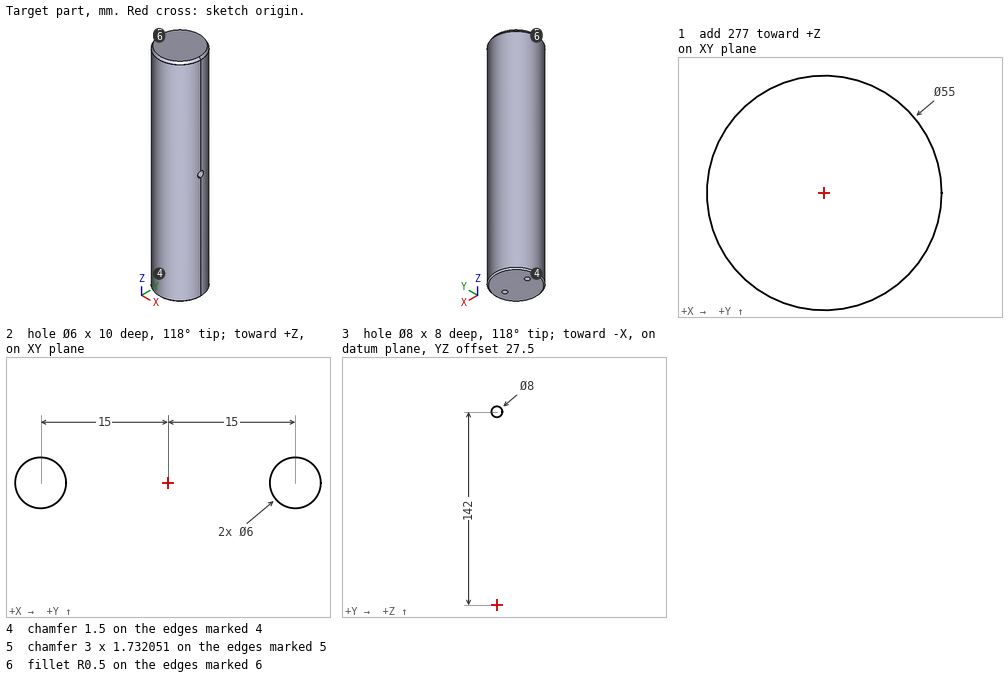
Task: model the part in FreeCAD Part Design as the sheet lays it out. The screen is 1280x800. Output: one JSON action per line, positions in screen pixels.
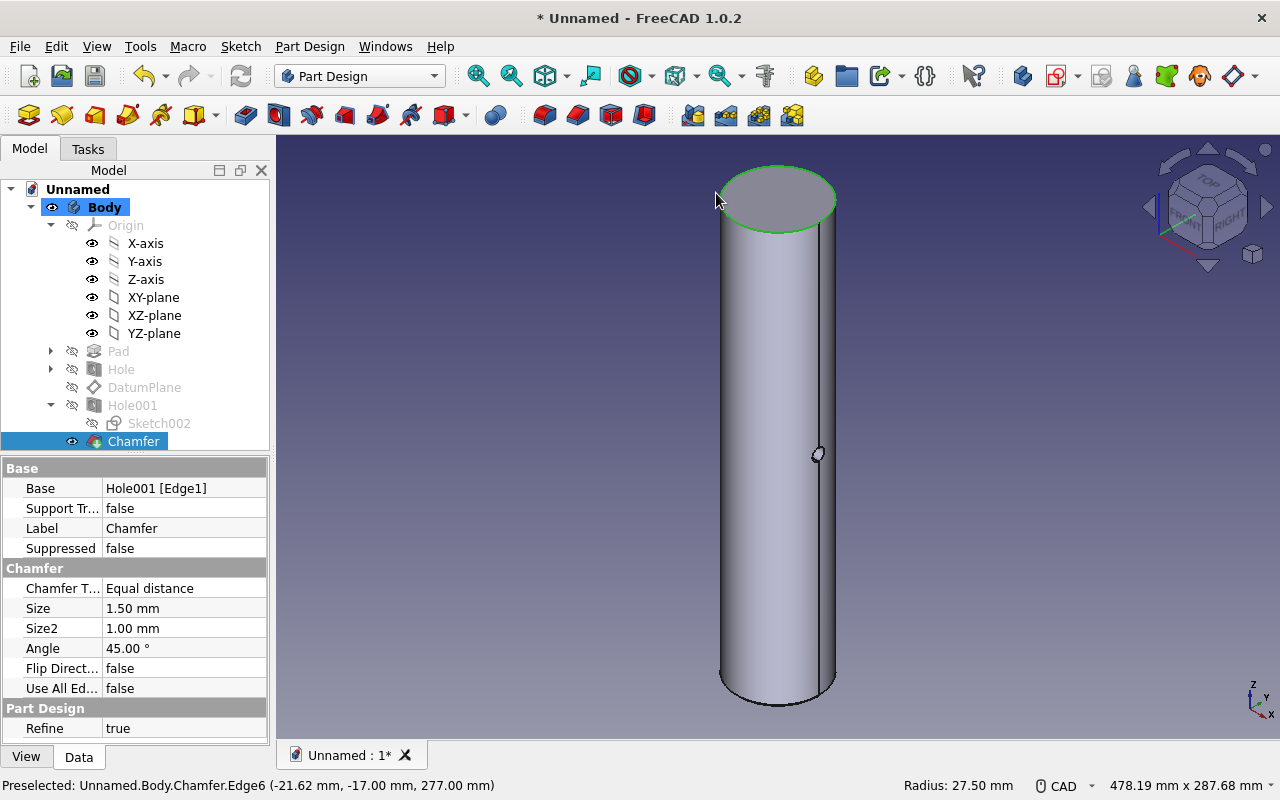
{"action": "left_click", "coordinate": [578, 116]}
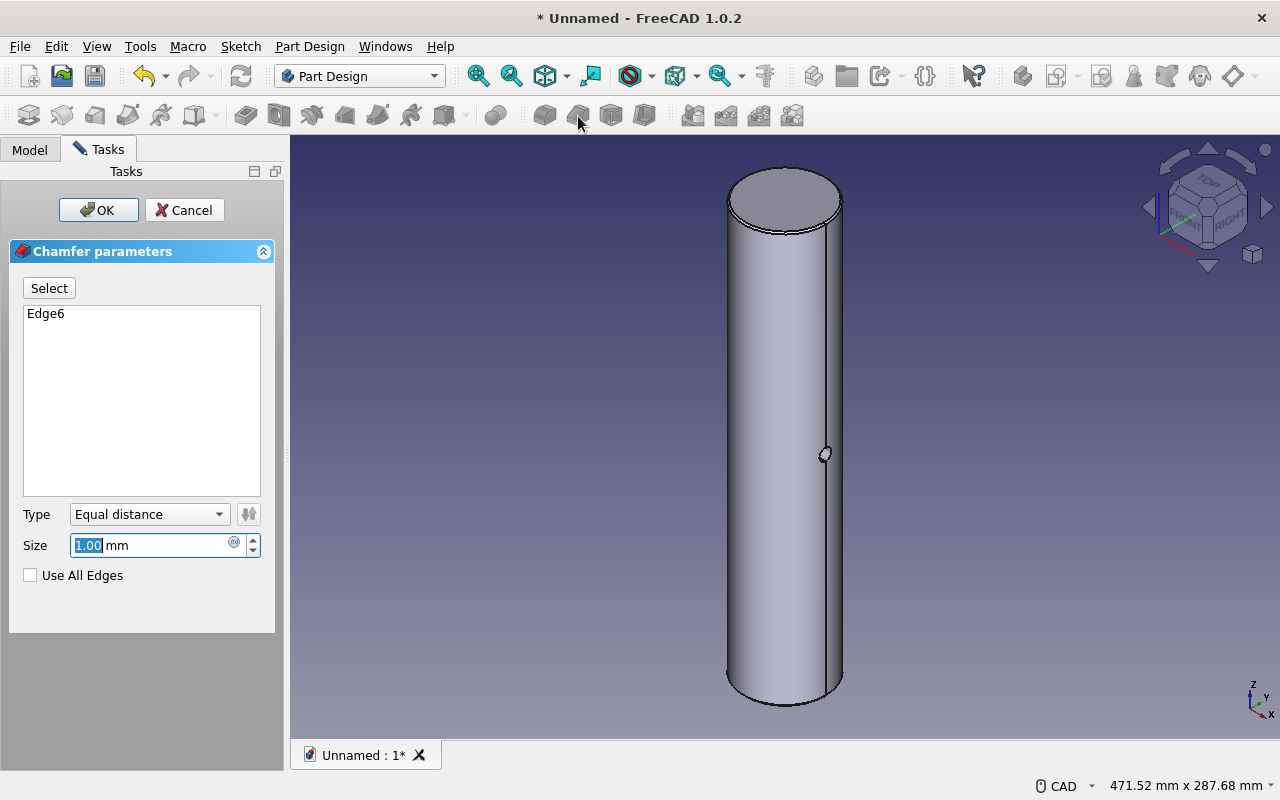
{"action": "type", "text": "3"}
{"action": "key", "text": "Tab"}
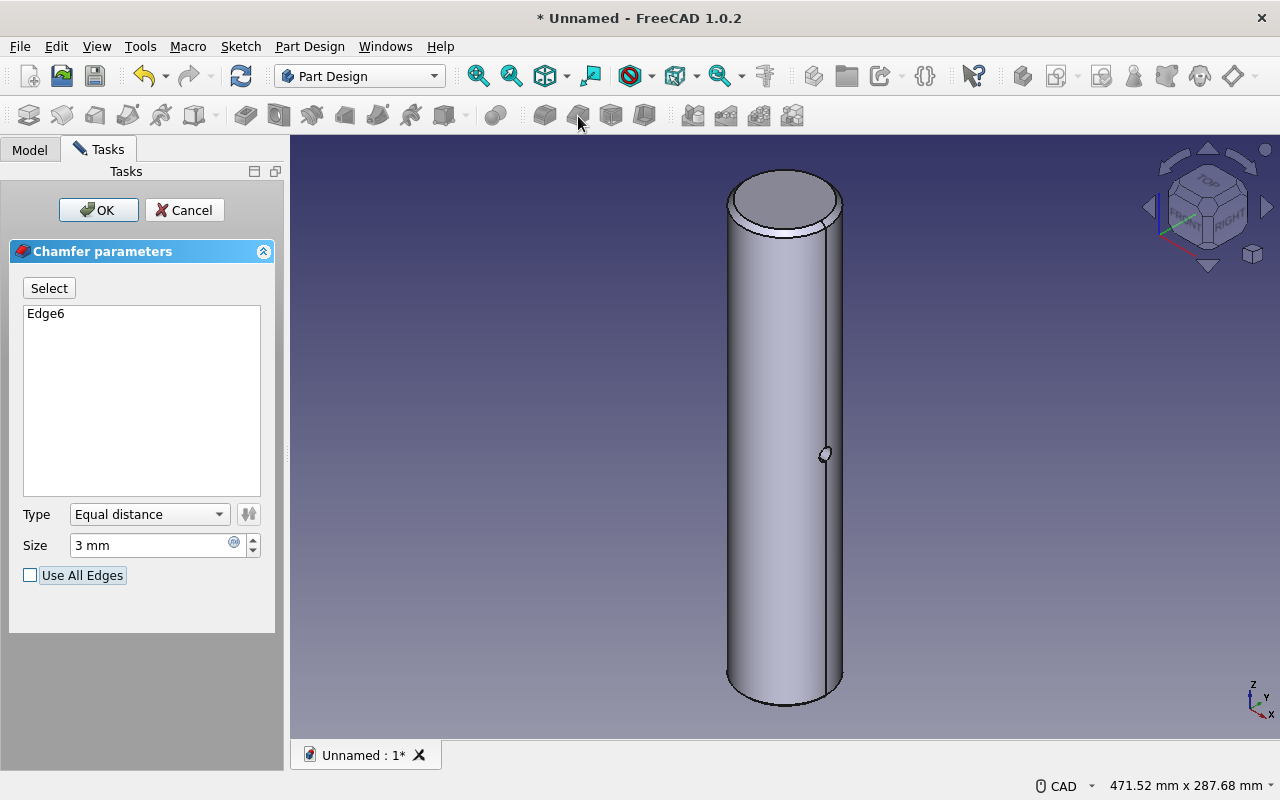
{"action": "left_click", "coordinate": [150, 514]}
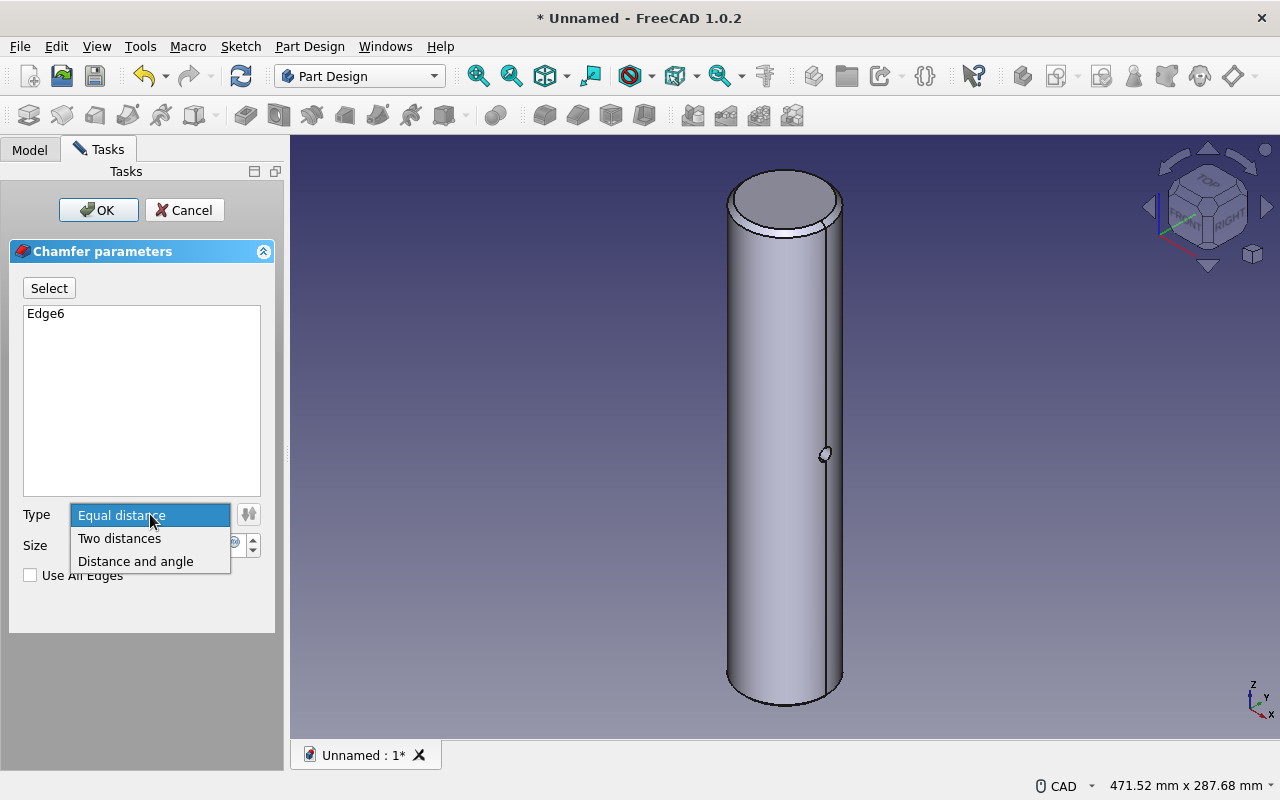
{"action": "left_click", "coordinate": [148, 538]}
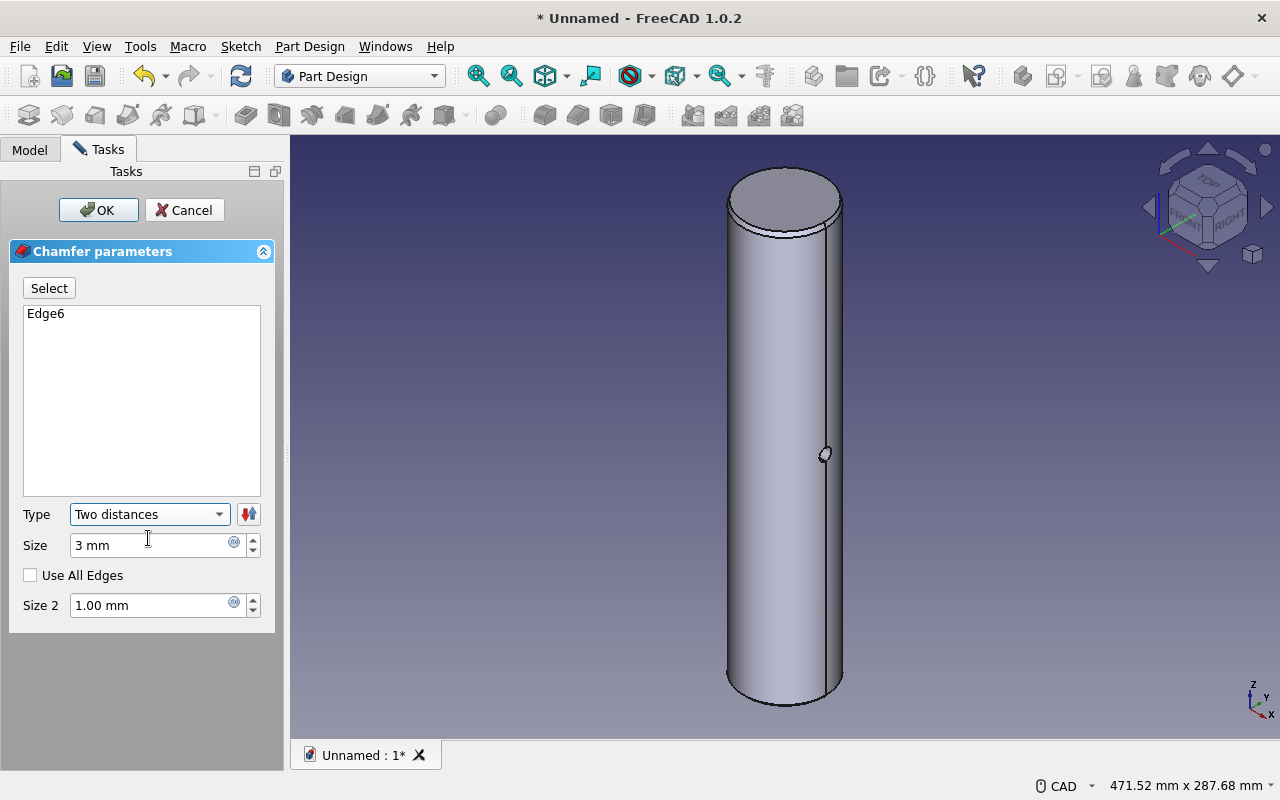
{"action": "triple_click", "coordinate": [158, 606]}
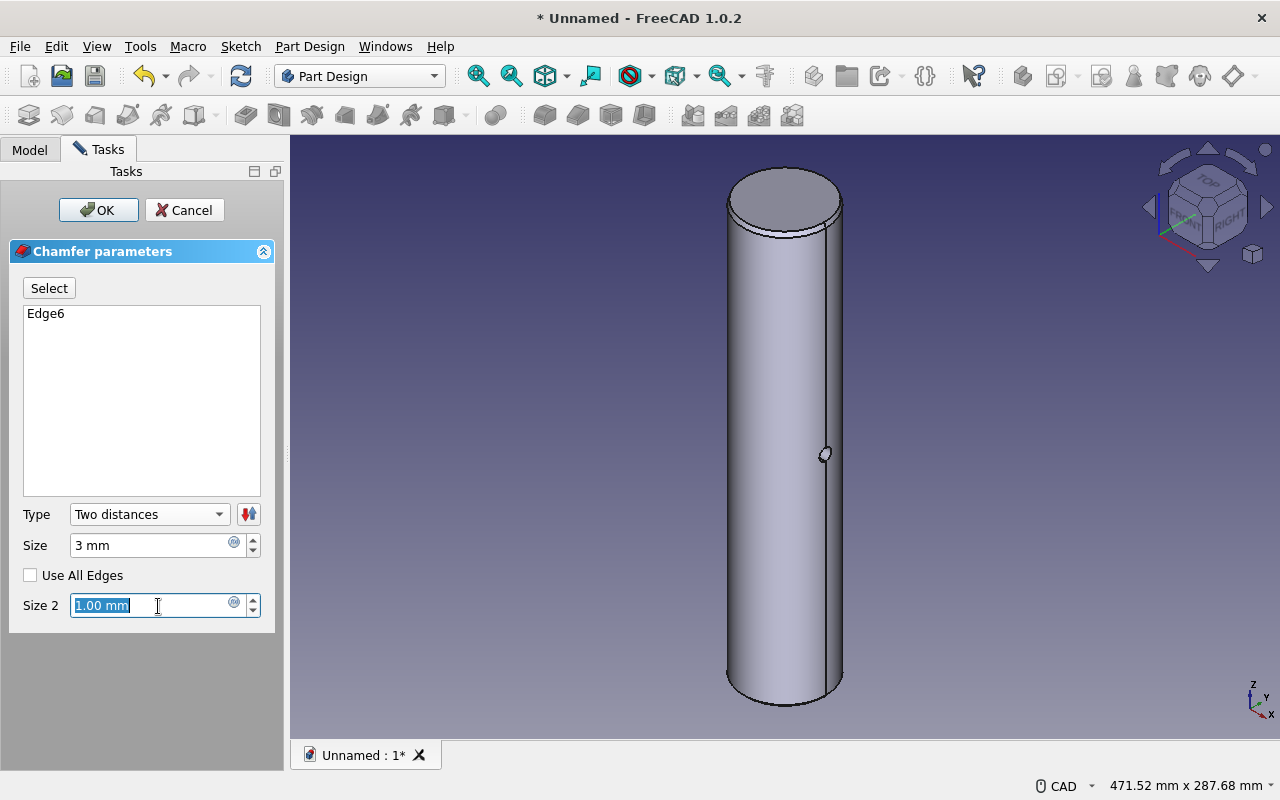
{"action": "type", "text": "1.732051"}
{"action": "key", "text": "Tab"}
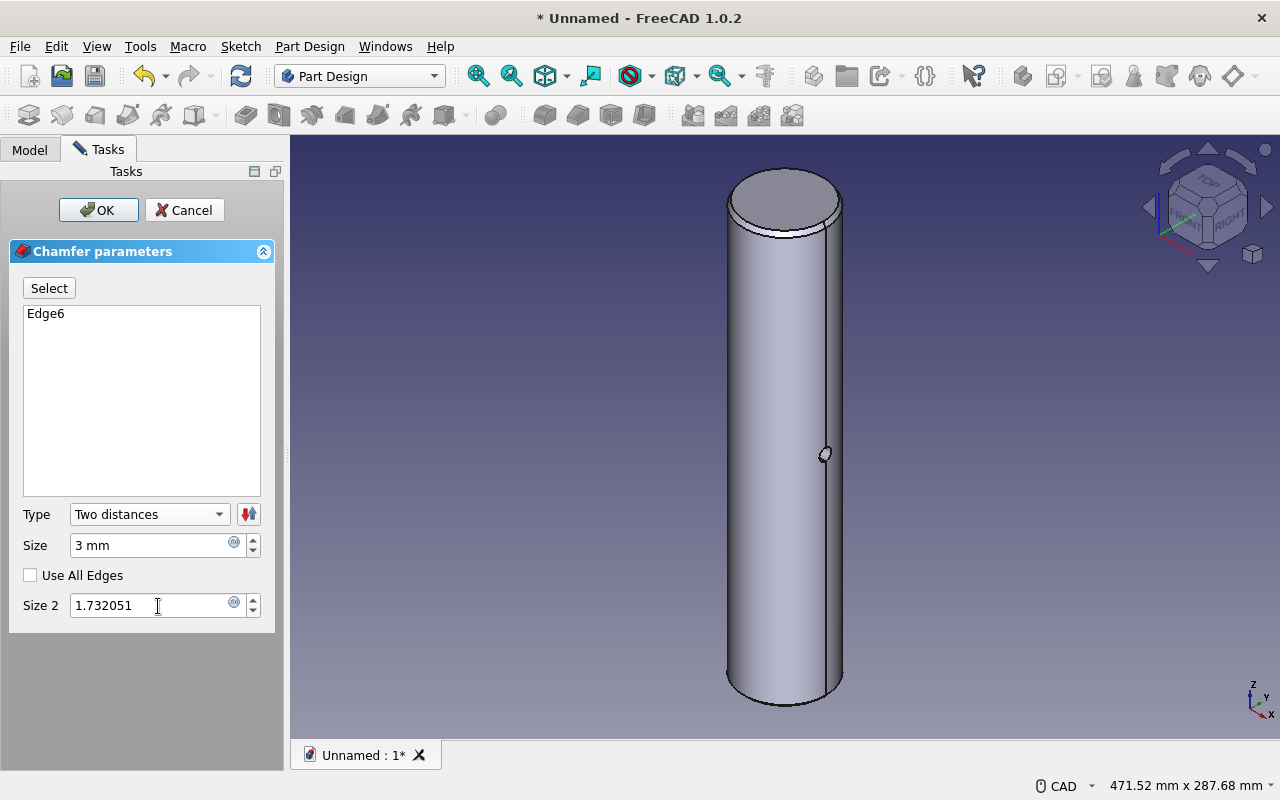
{"action": "left_click", "coordinate": [99, 210]}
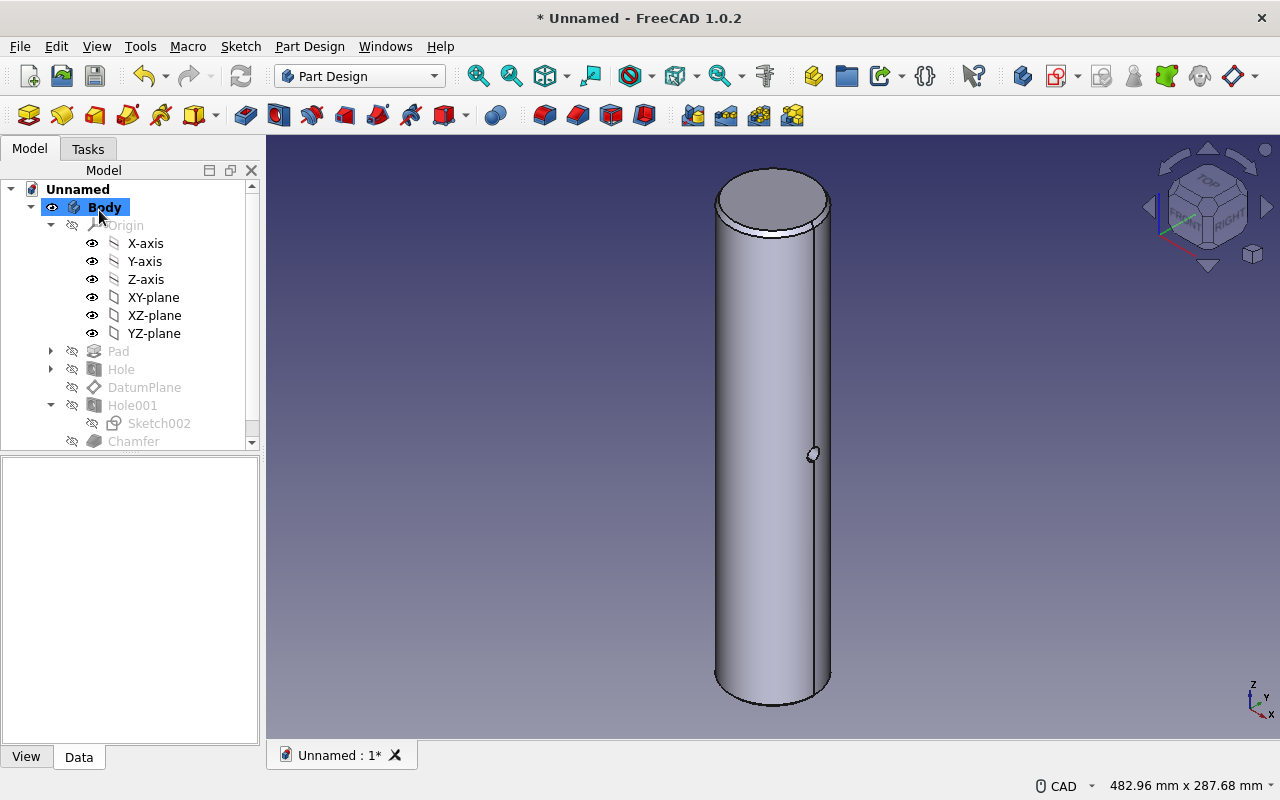
{"action": "key", "text": "2"}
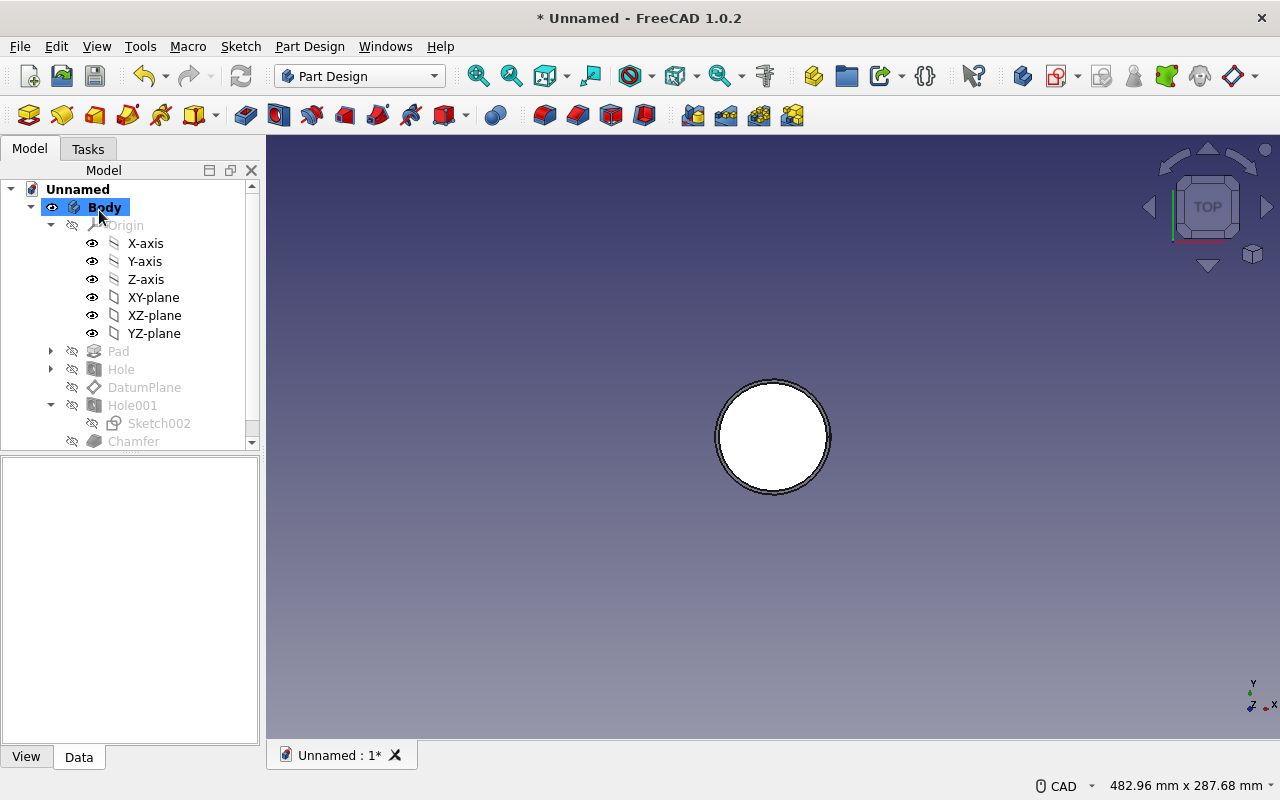
{"action": "key", "text": "v f"}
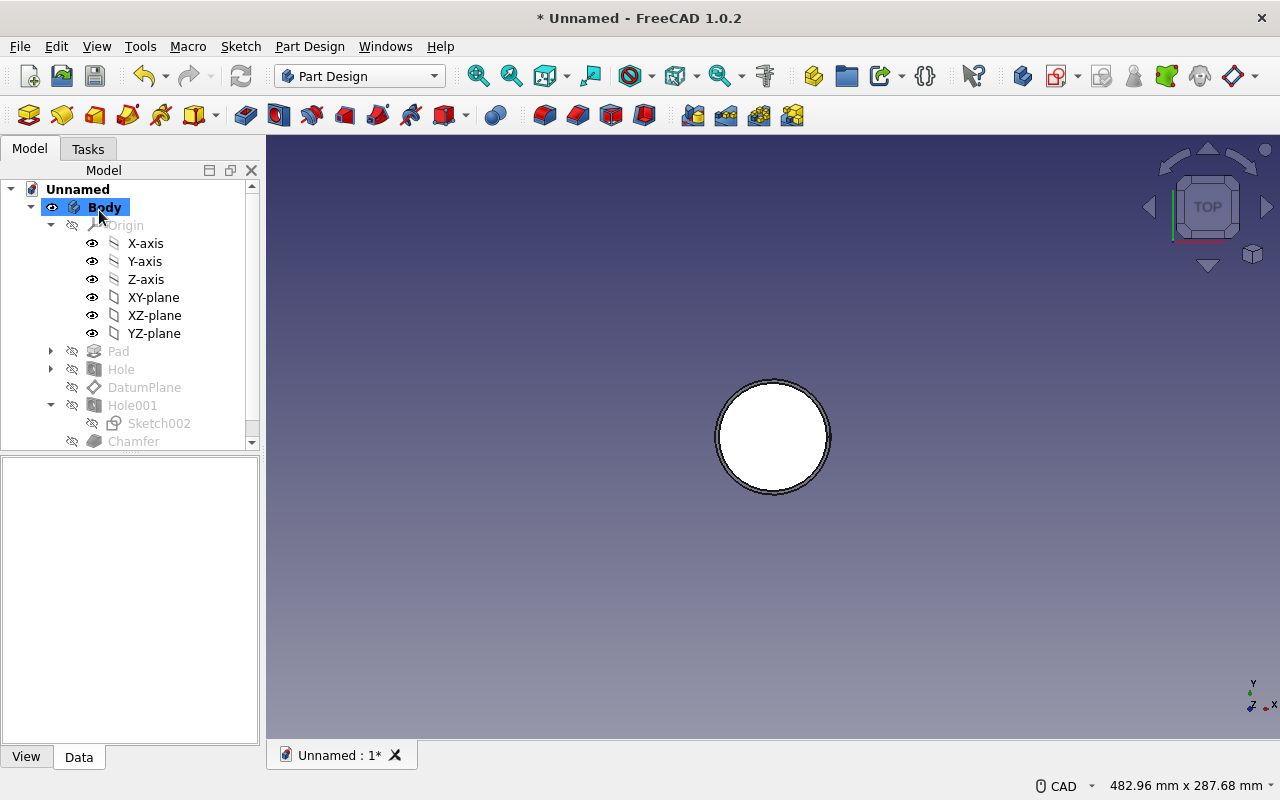
{"action": "key", "text": "0"}